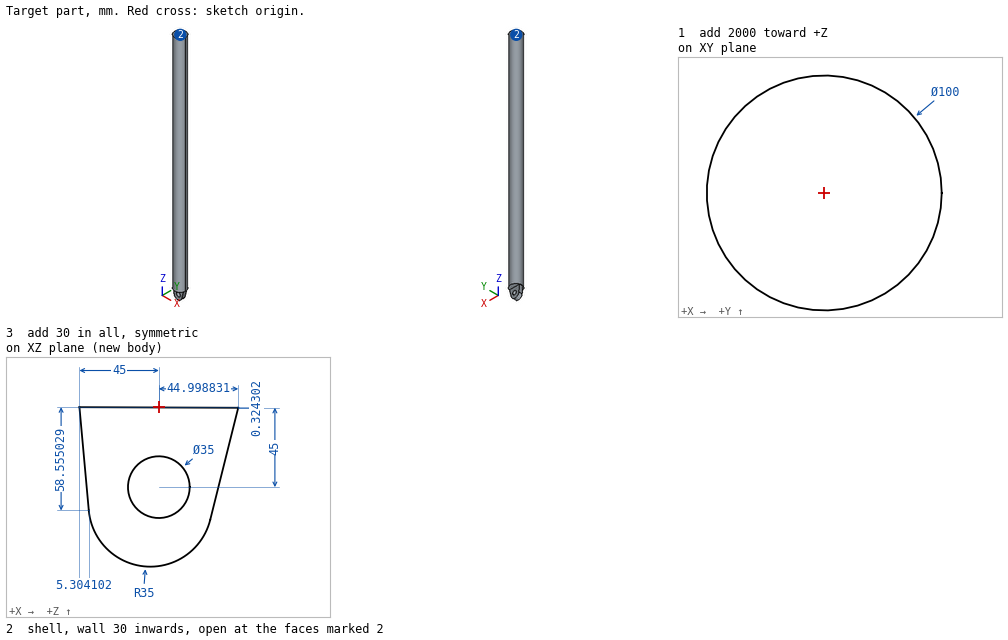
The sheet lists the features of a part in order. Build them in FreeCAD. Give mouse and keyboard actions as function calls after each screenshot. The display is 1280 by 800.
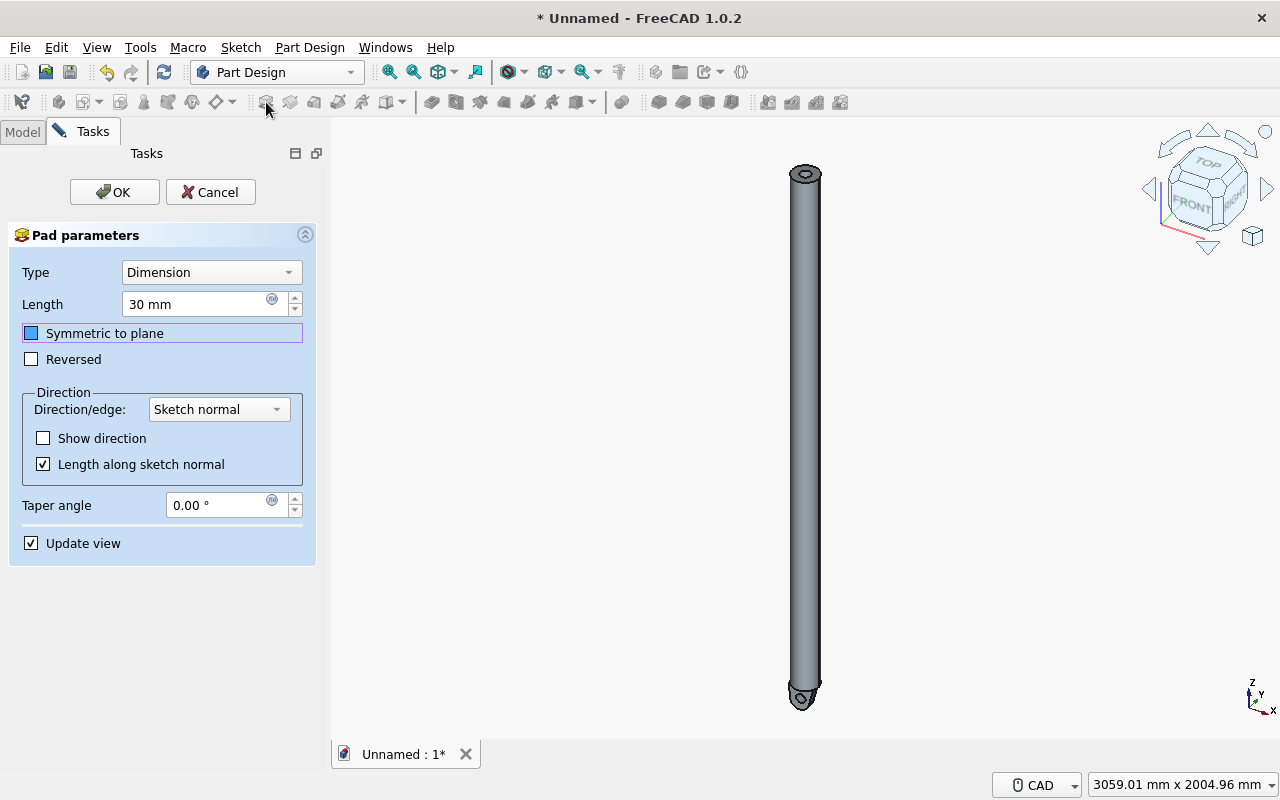
click(30, 333)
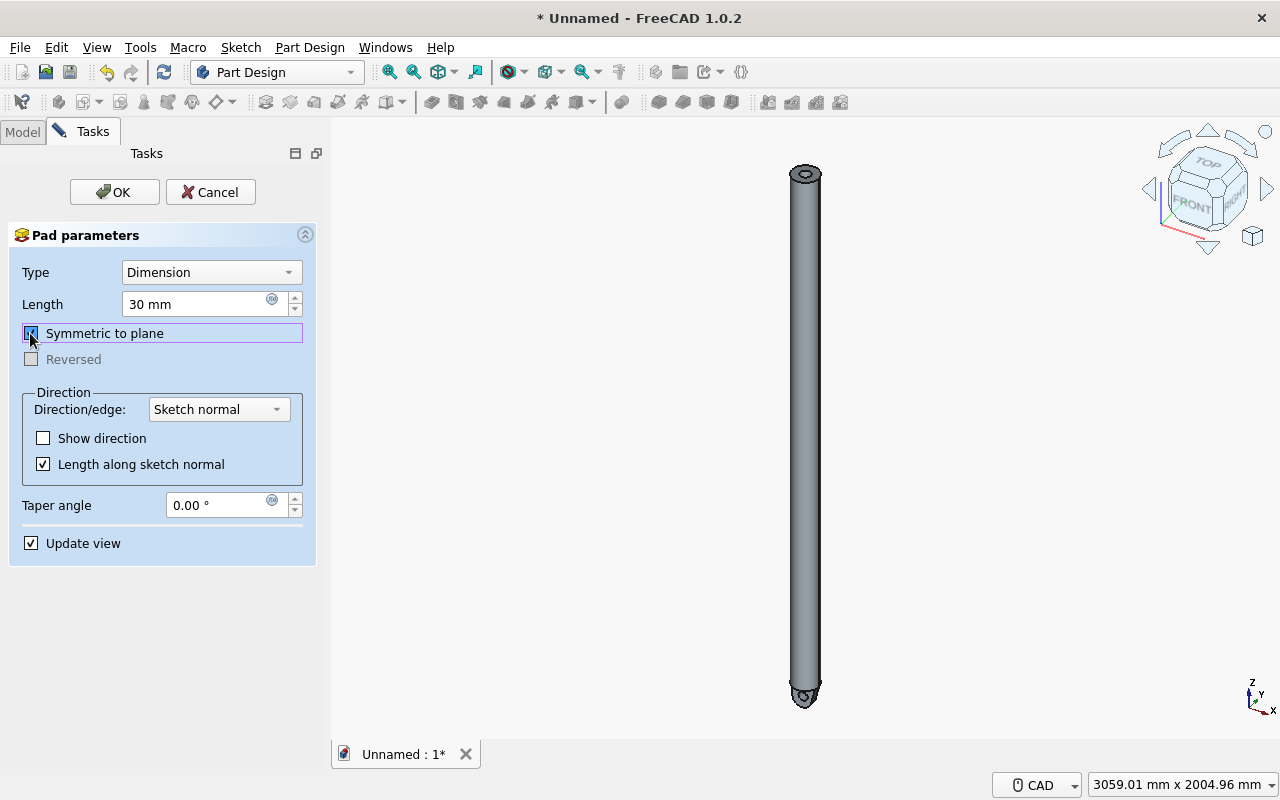
click(115, 192)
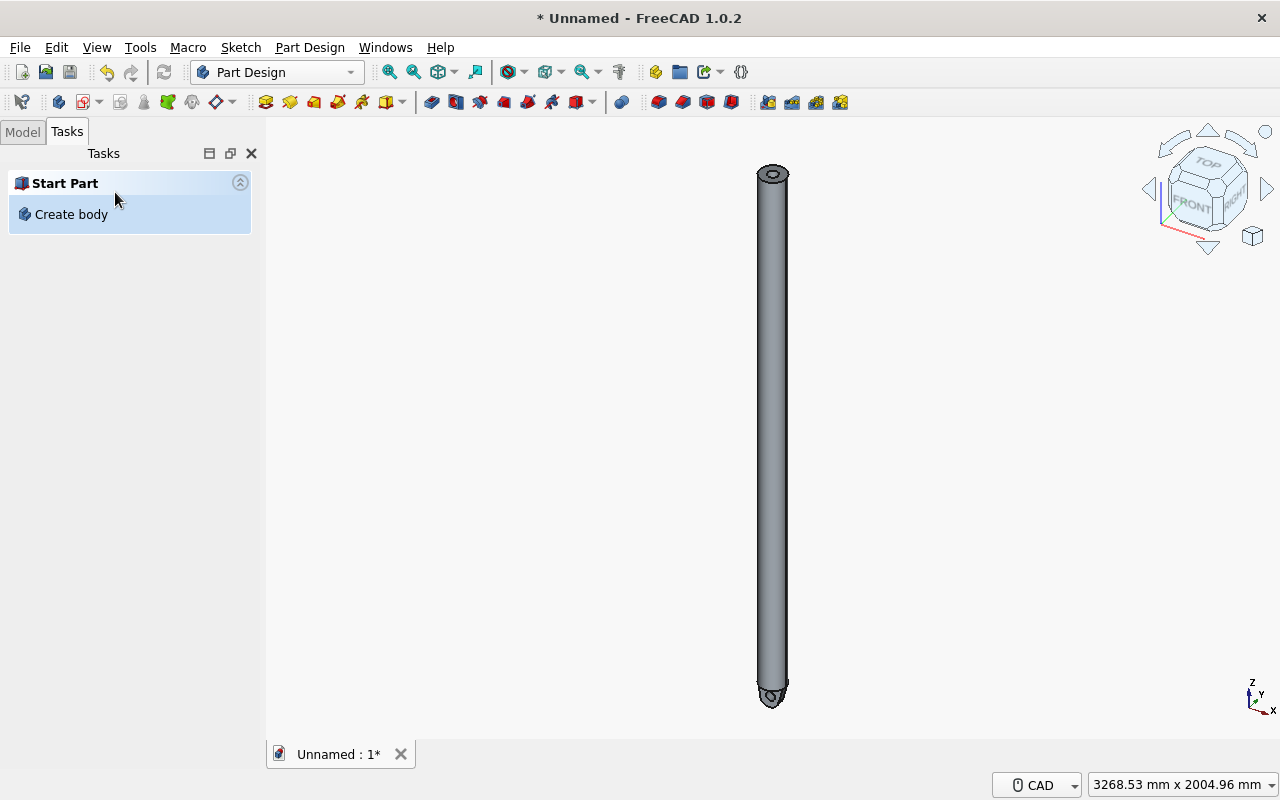
key(0)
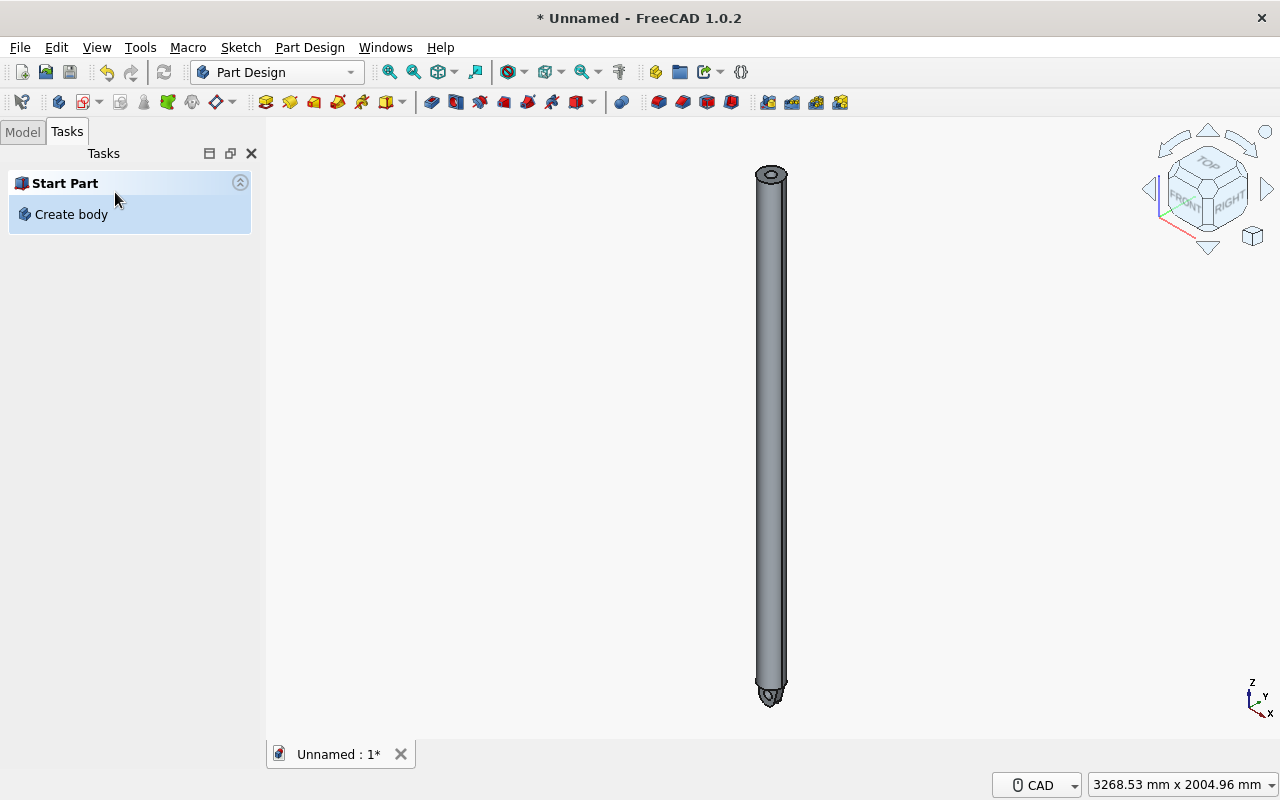
key(v)
key(f)